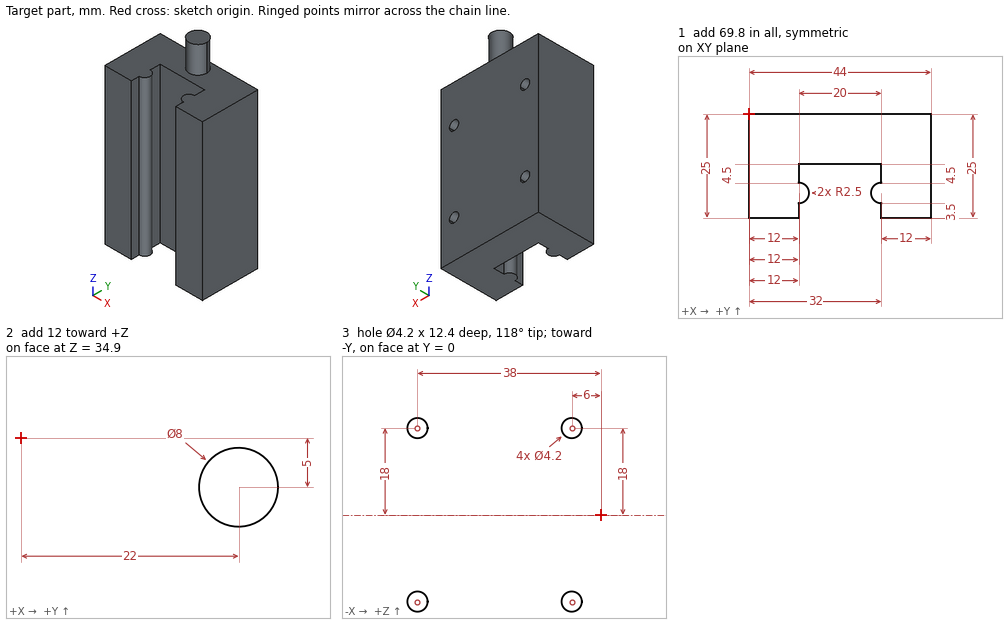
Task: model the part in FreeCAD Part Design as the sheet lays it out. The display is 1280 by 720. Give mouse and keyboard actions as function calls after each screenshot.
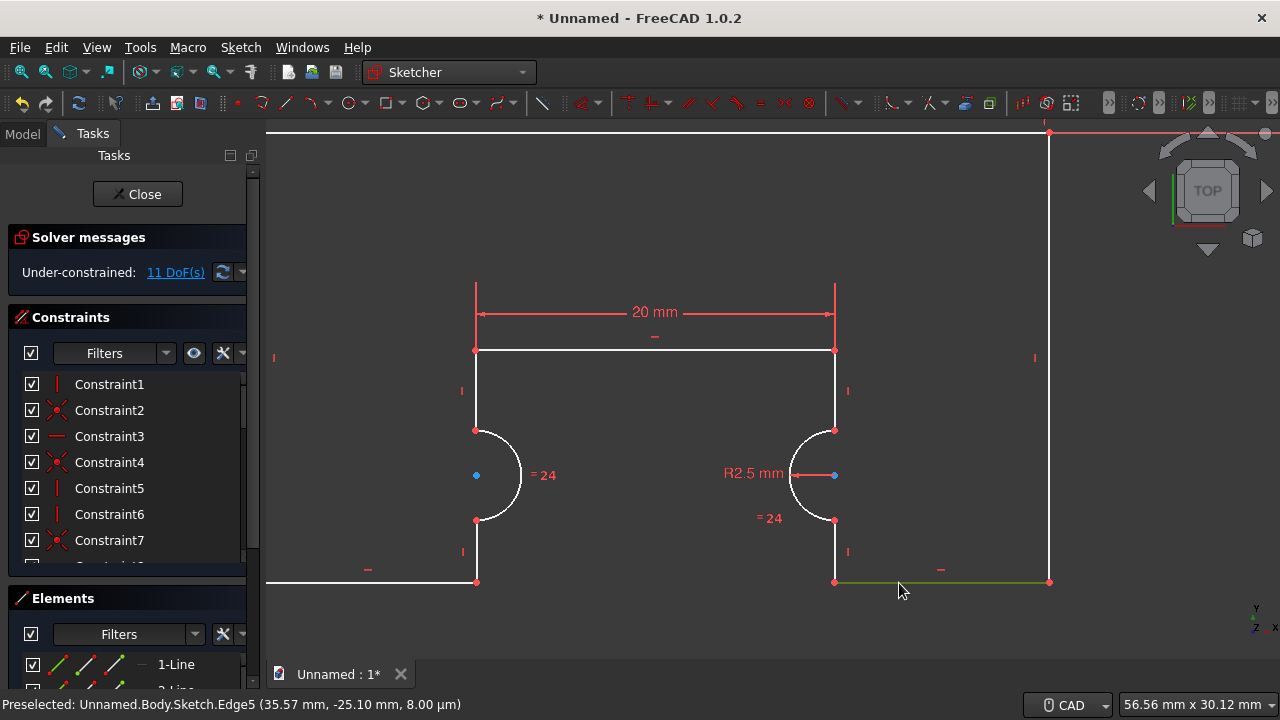
key(l)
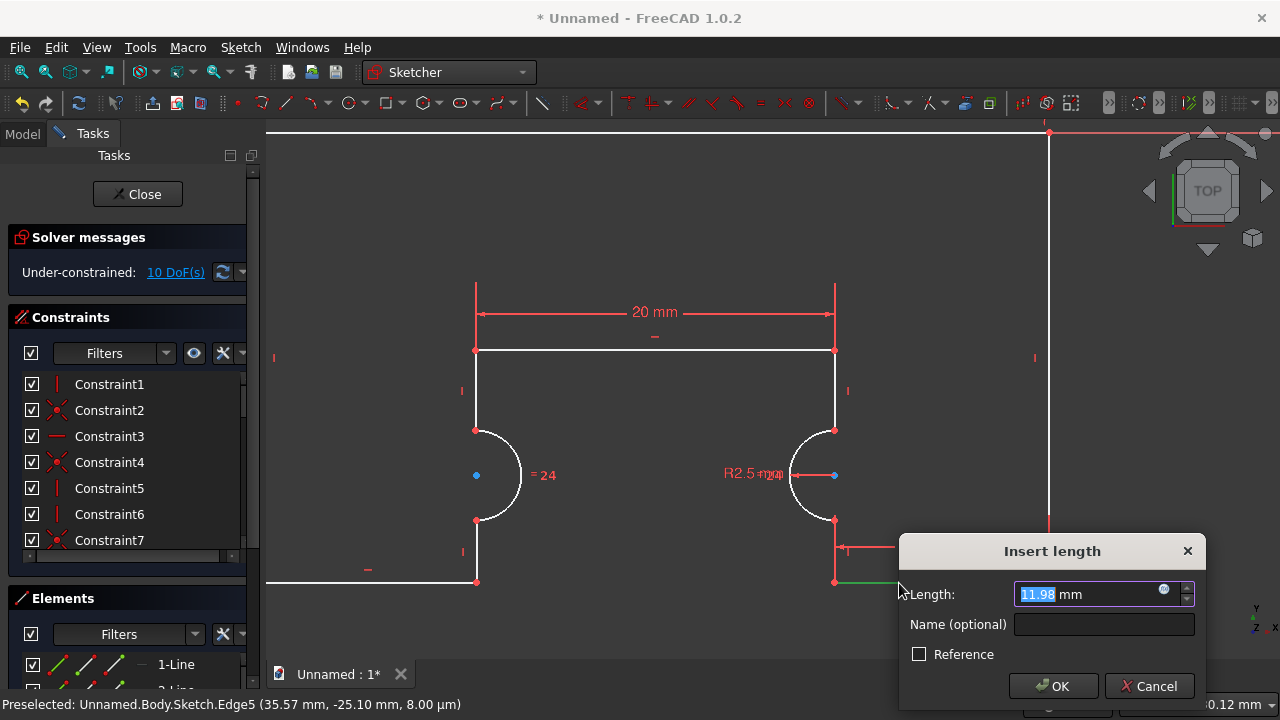
text(12)
key(Return)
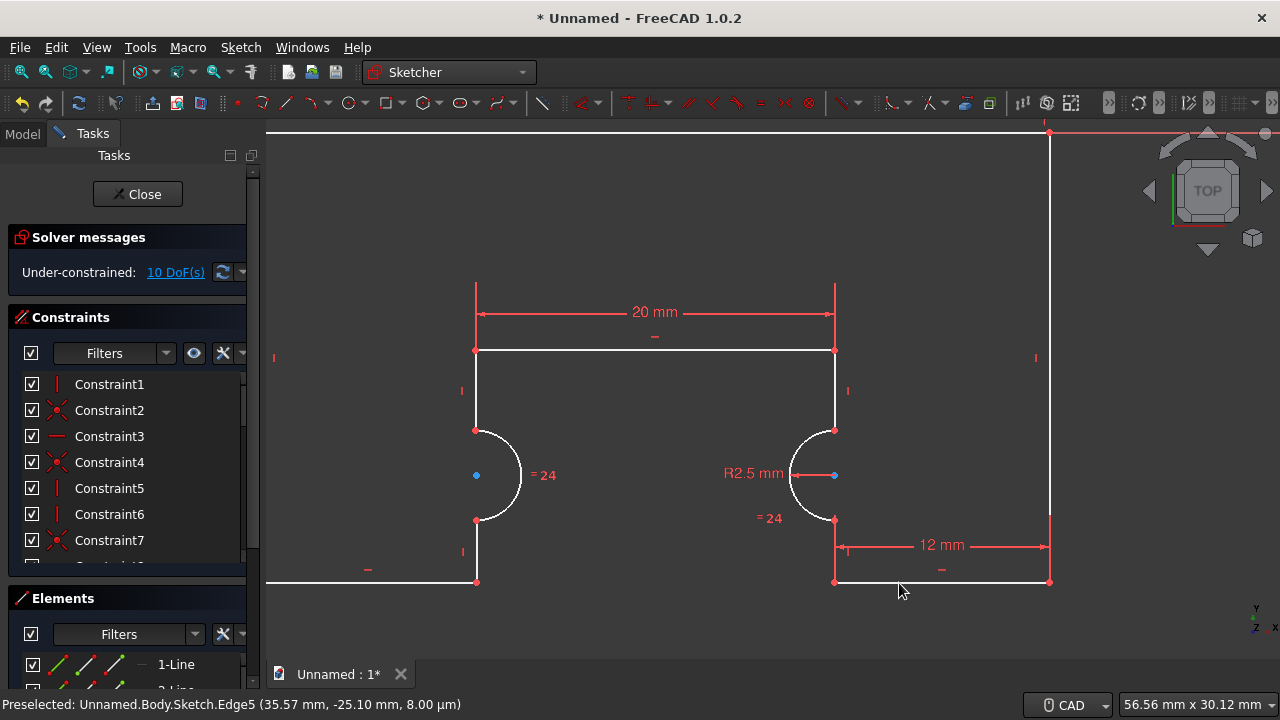
click(1050, 448)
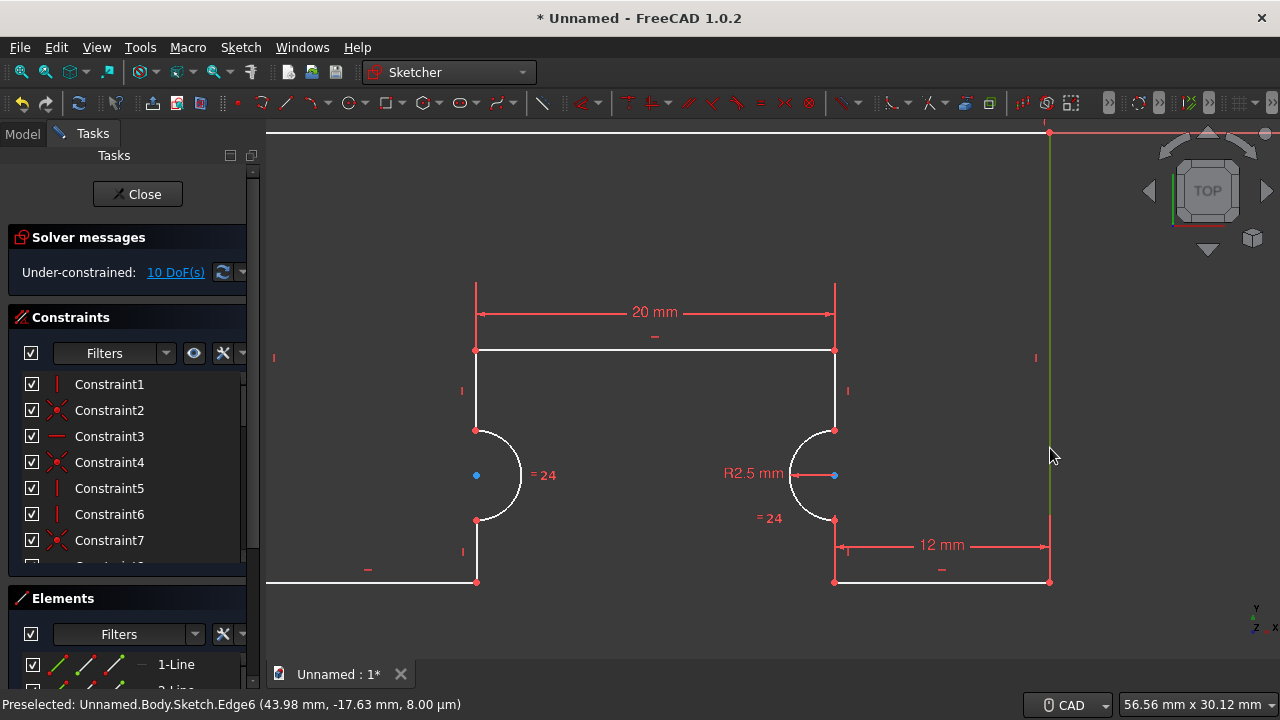
click(600, 104)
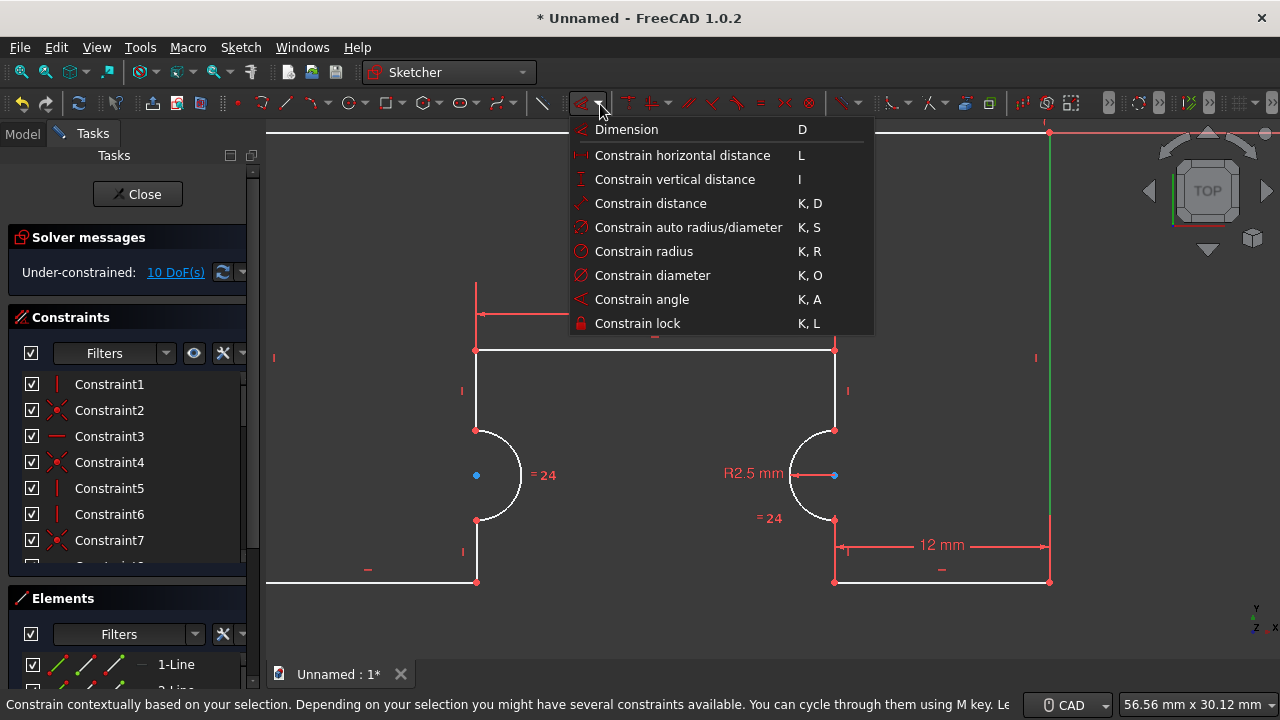
click(722, 179)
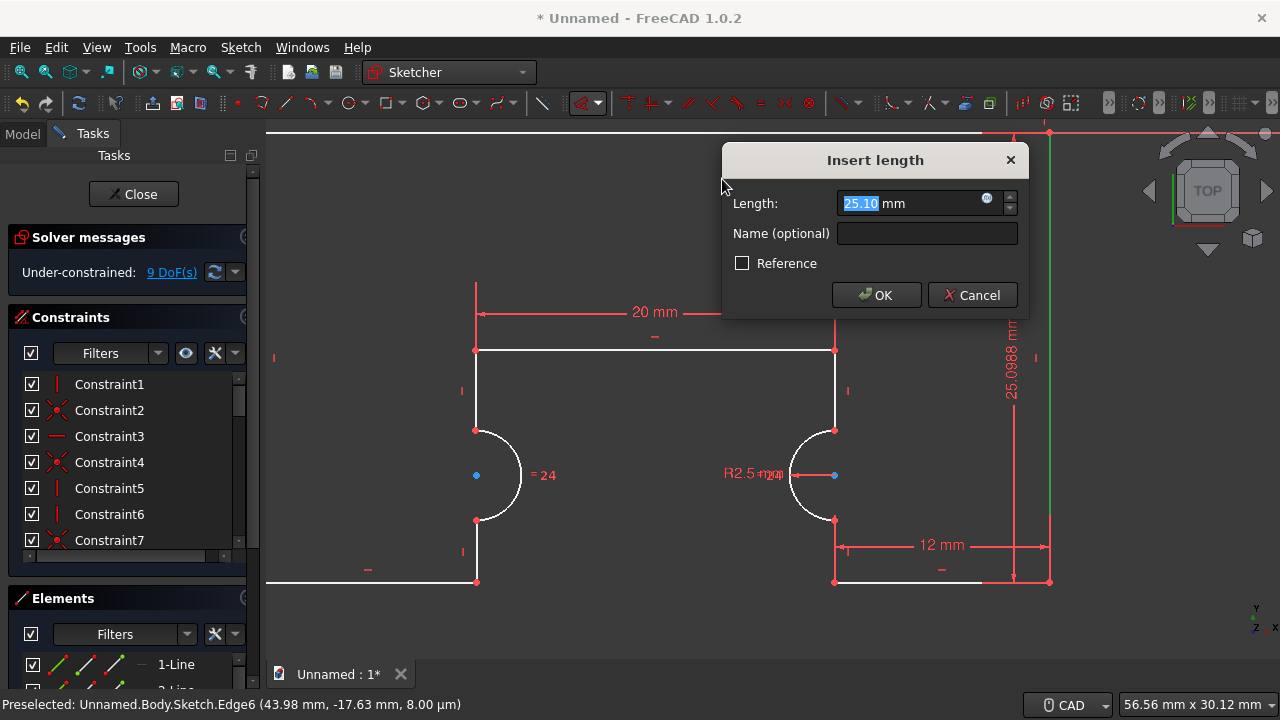
text(25)
key(Return)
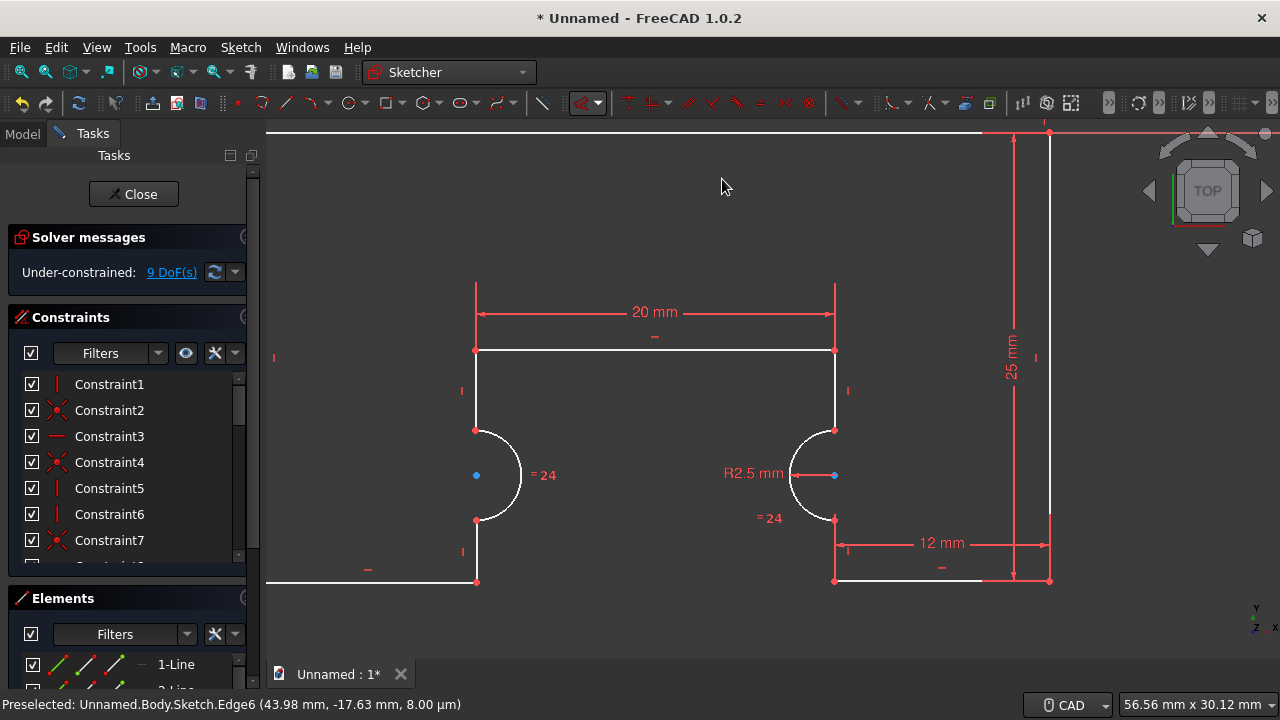
scroll(804, 454, down, 2)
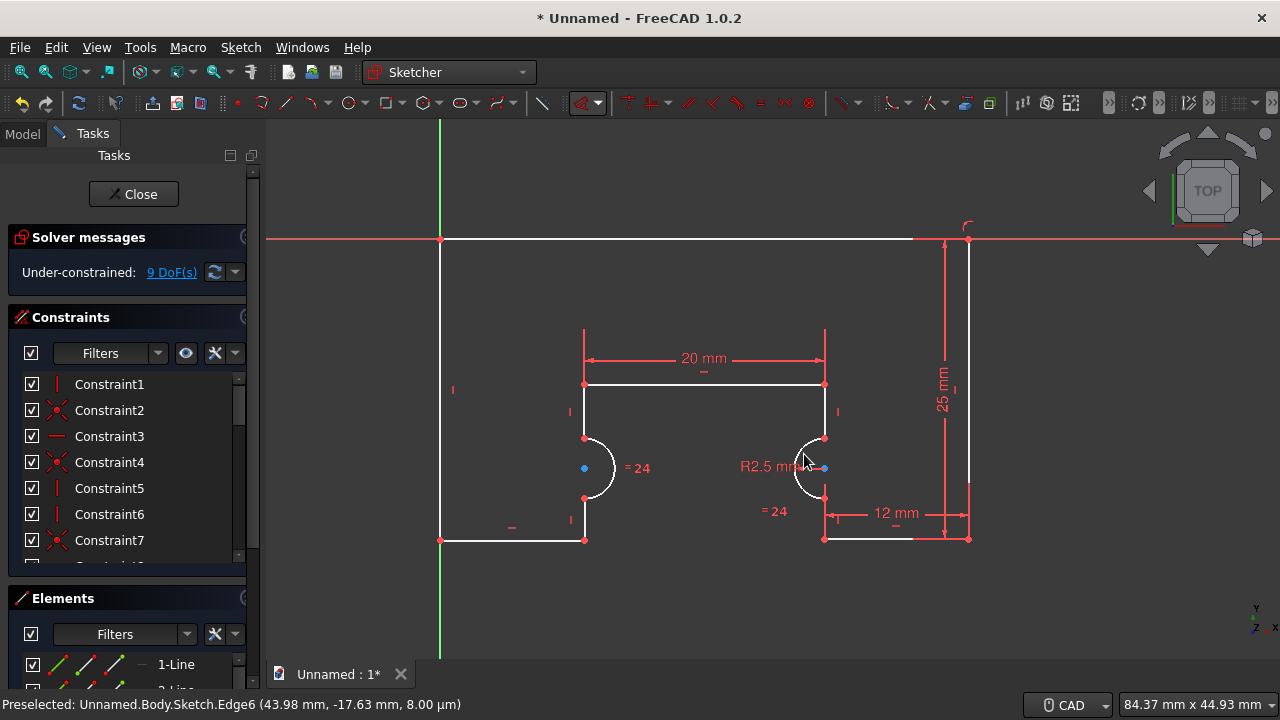
click(810, 239)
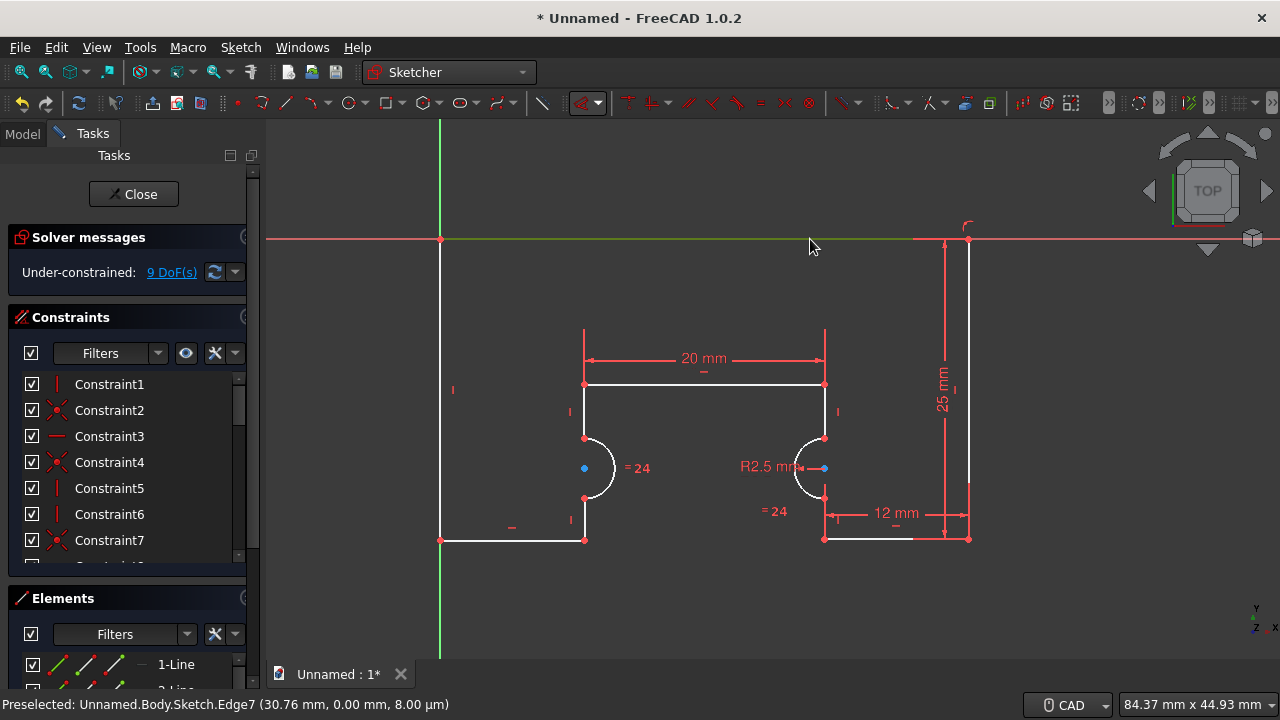
key(l)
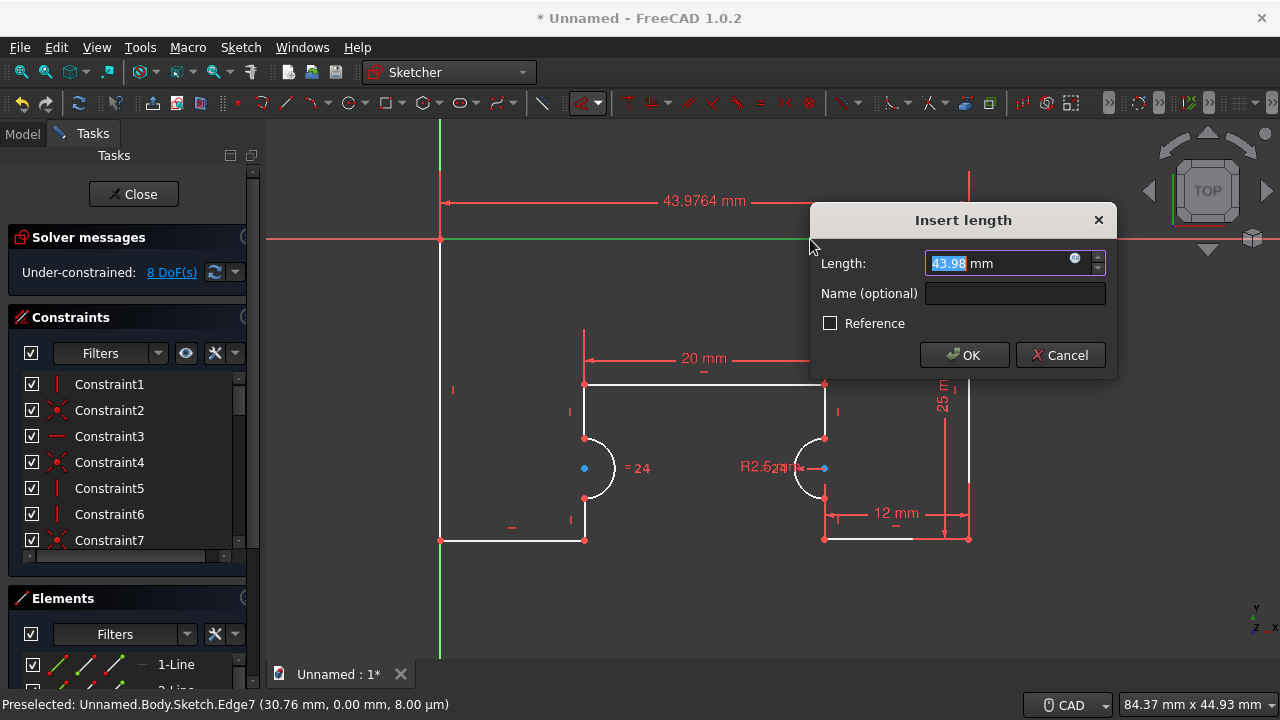
text(44)
key(Return)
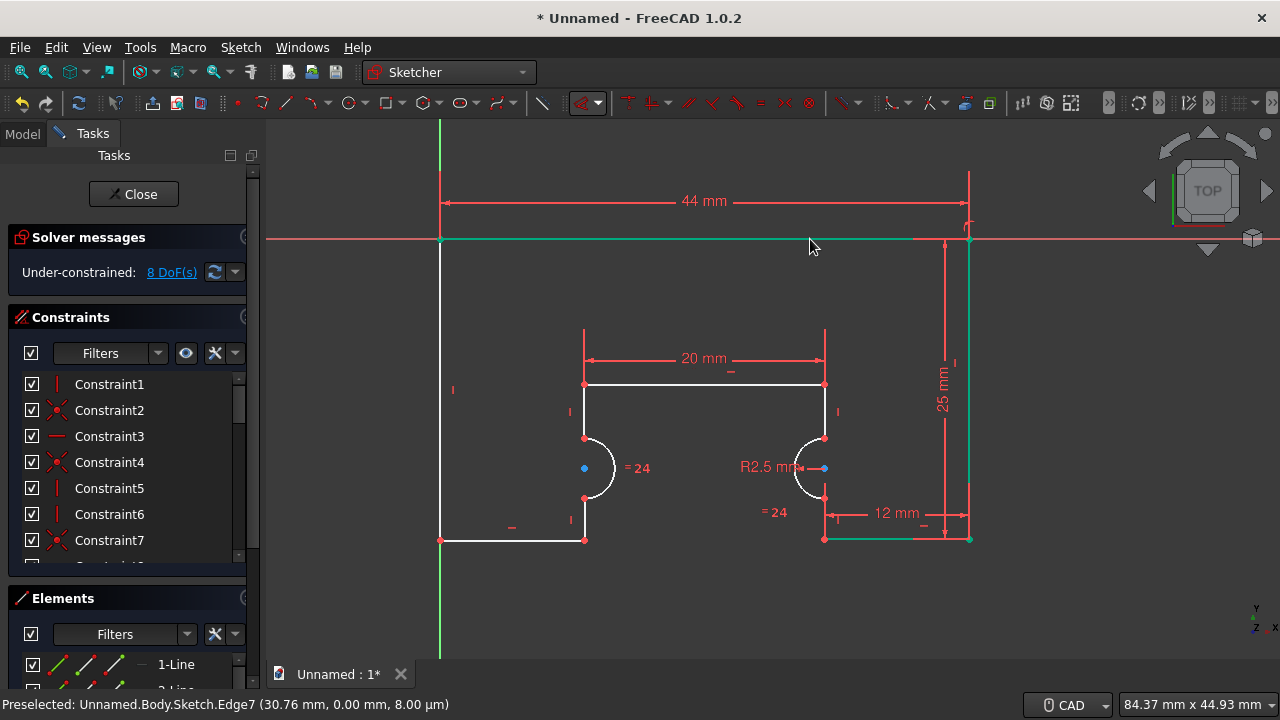
click(440, 330)